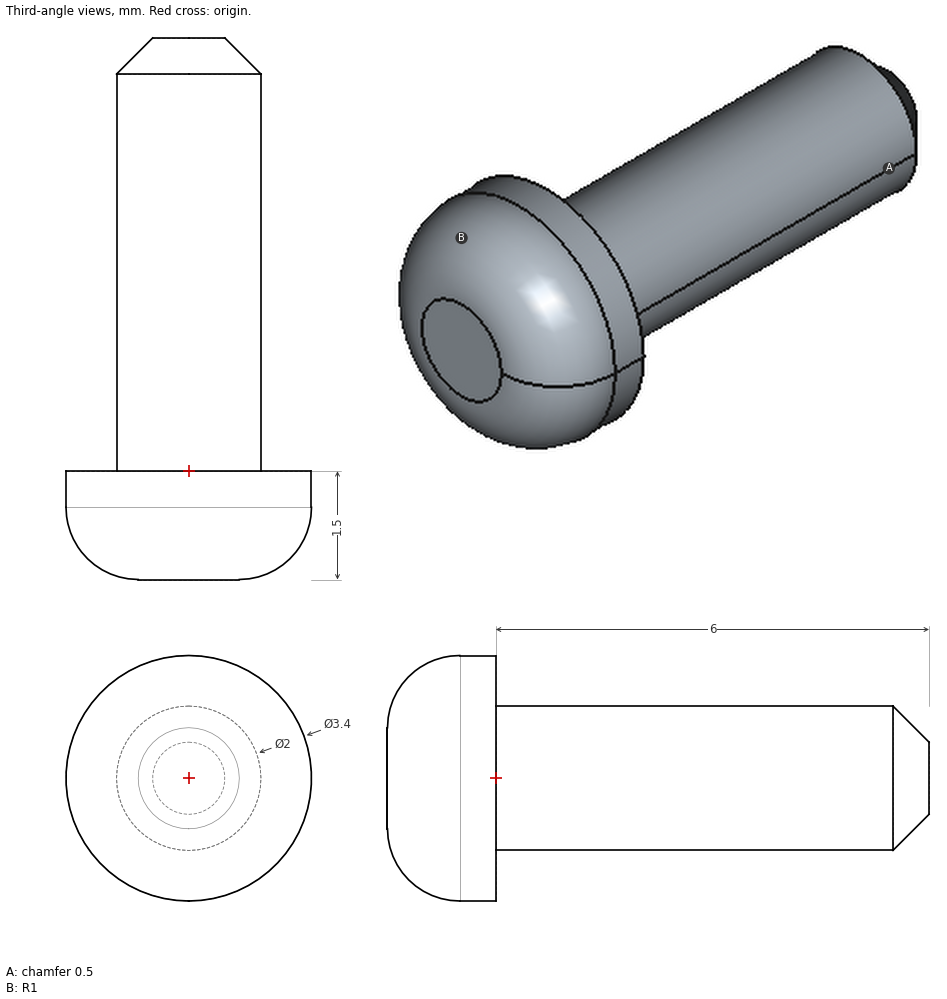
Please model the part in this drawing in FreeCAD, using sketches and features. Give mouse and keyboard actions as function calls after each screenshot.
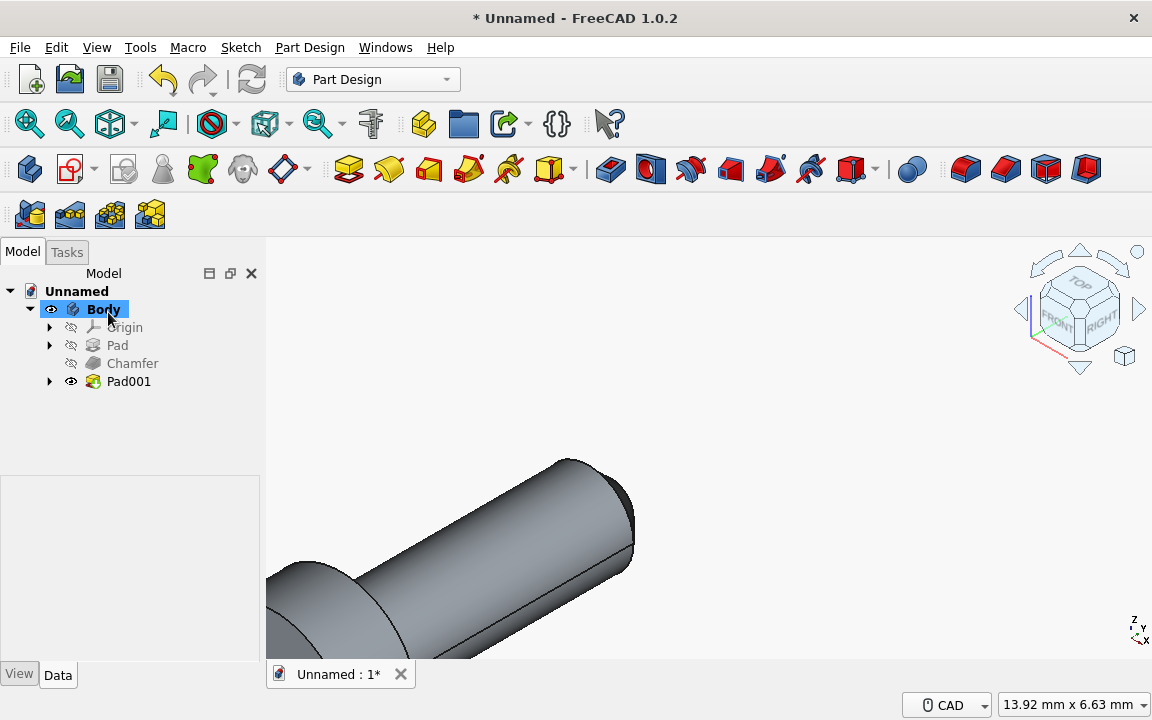
click(30, 124)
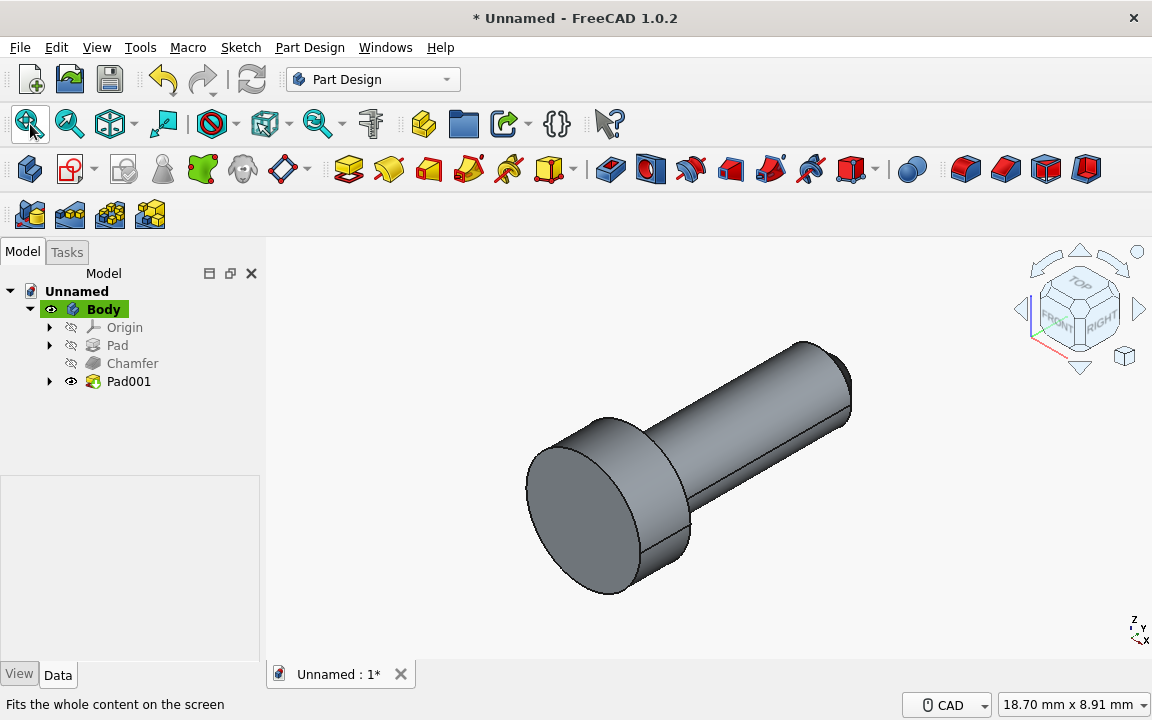
click(566, 447)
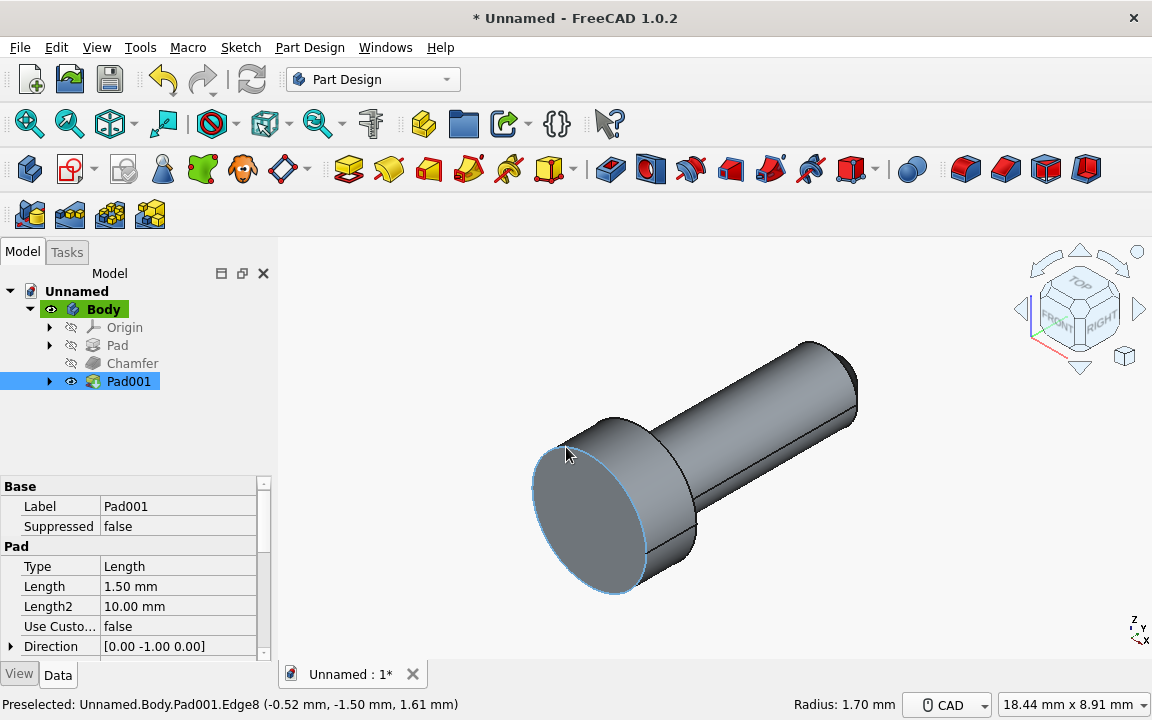
click(966, 170)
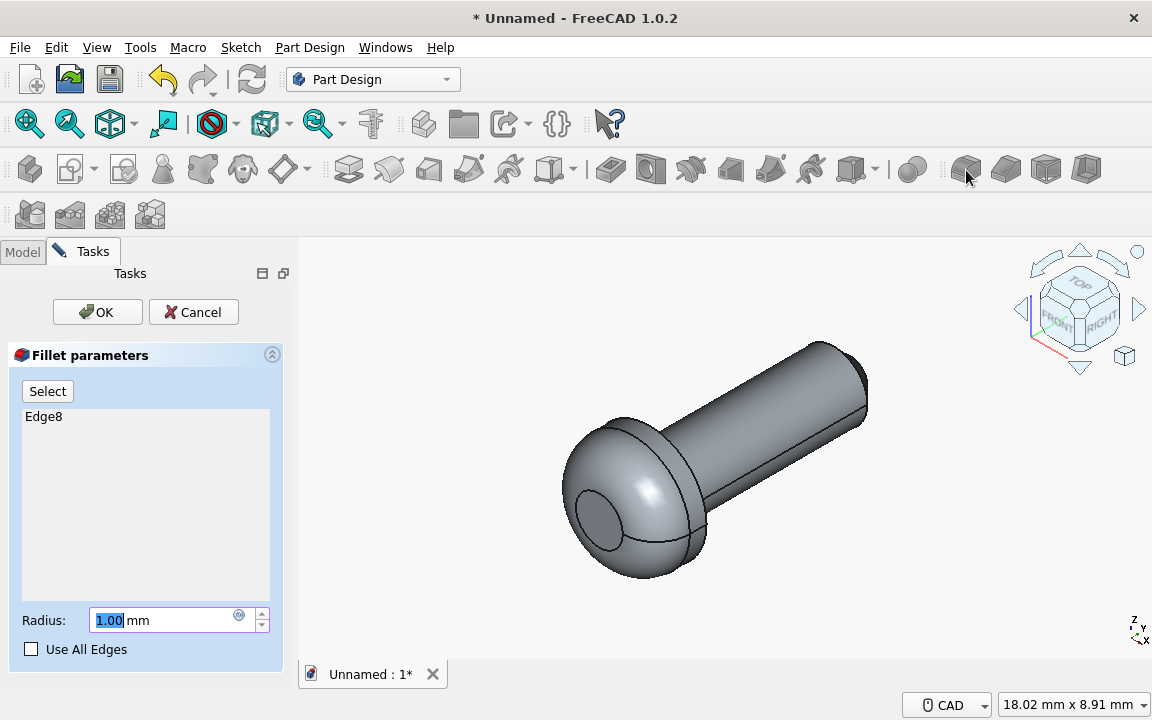
text(1)
key(Tab)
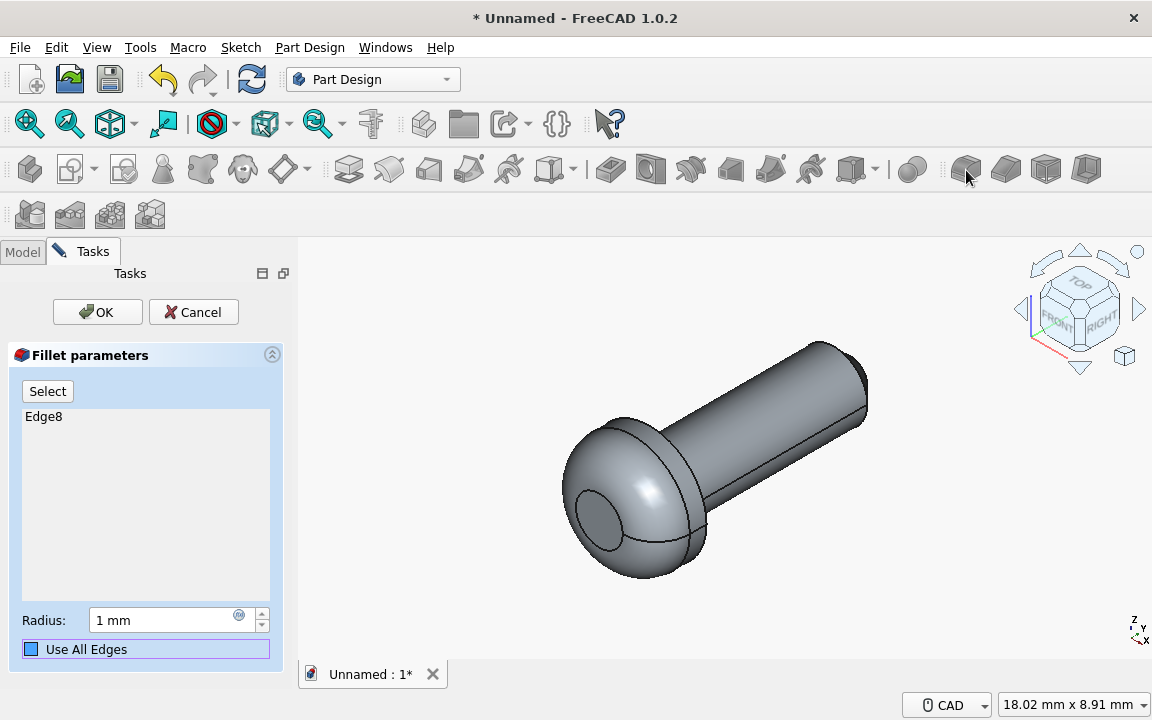
click(98, 312)